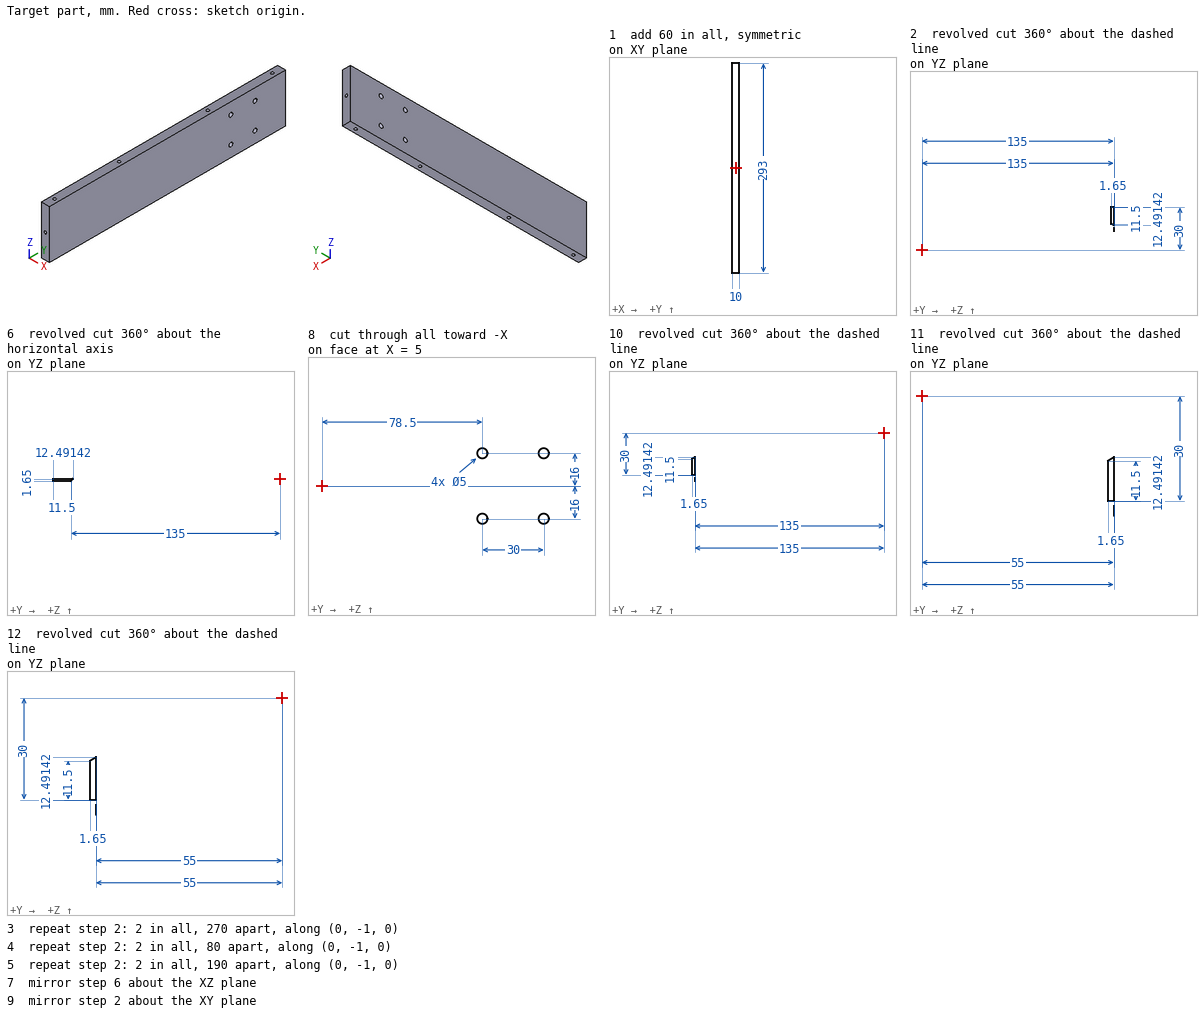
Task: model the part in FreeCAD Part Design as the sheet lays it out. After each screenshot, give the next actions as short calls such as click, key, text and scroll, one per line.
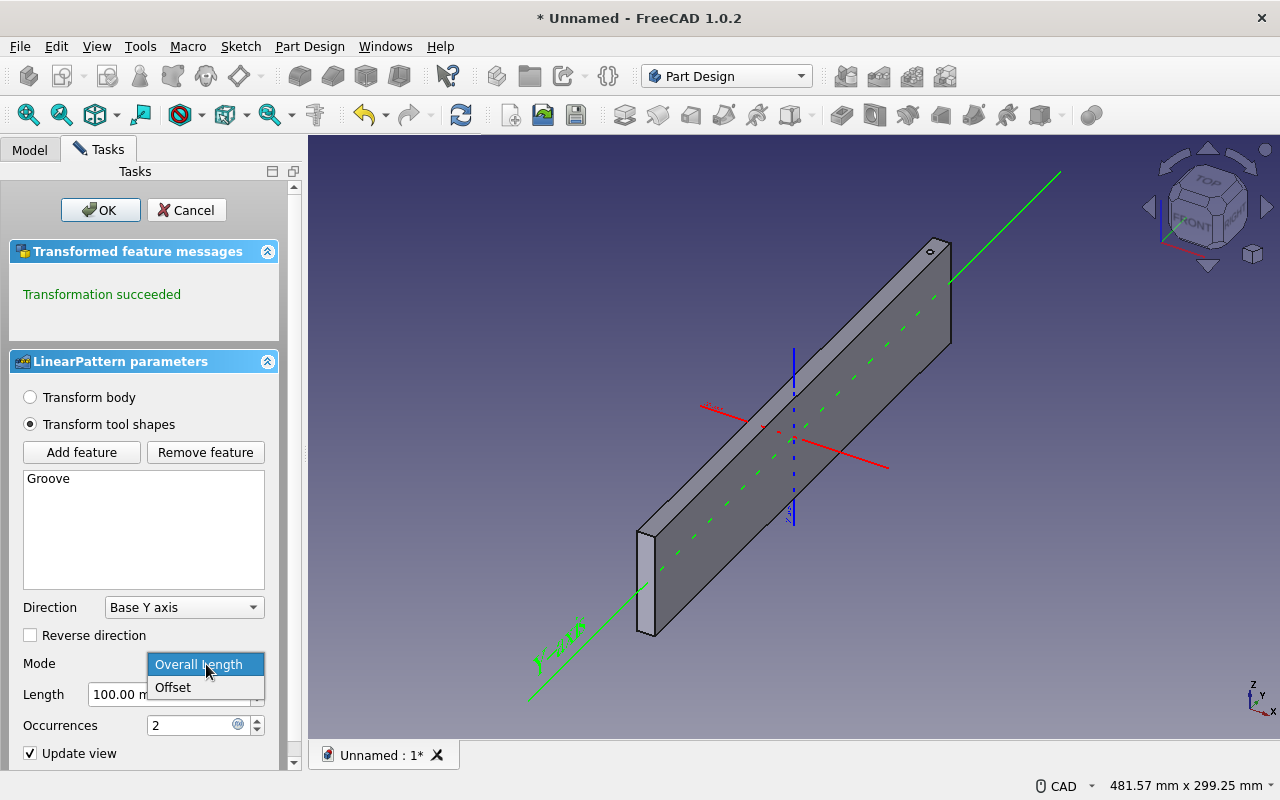
click(204, 688)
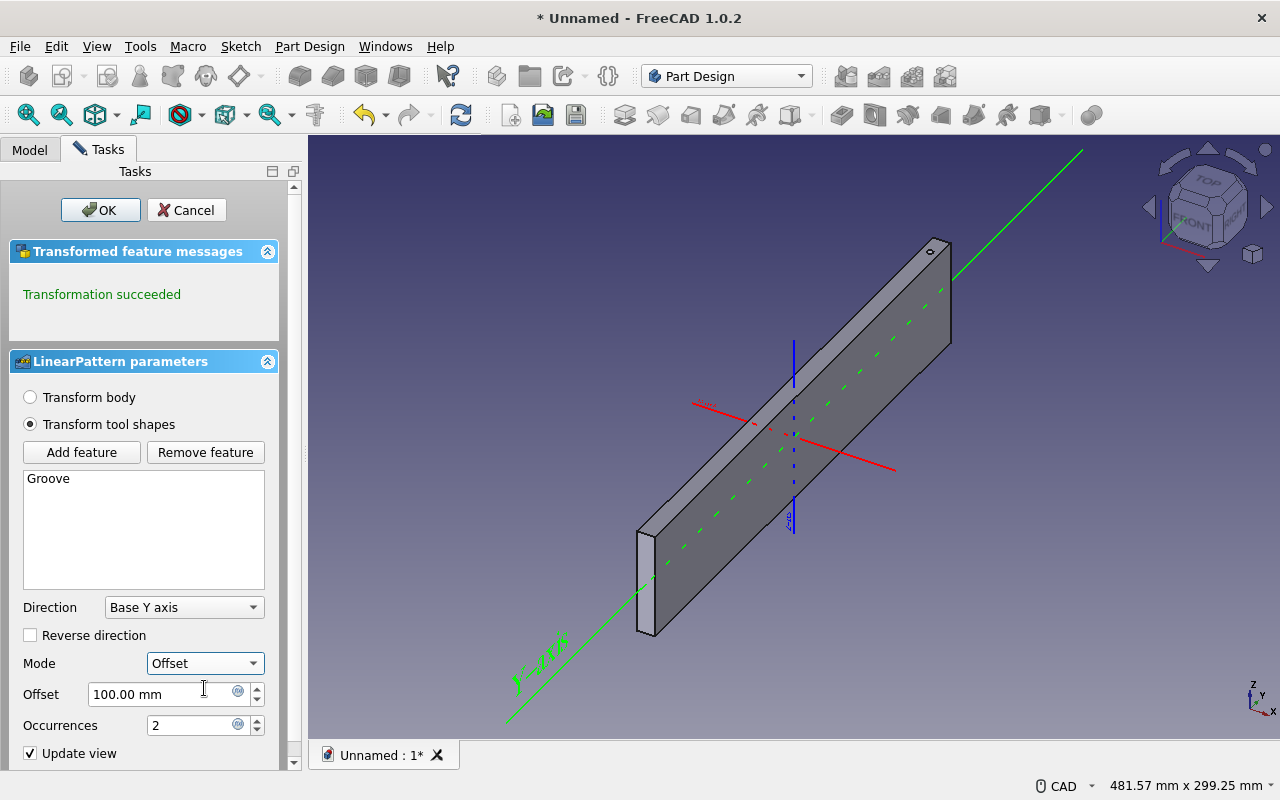
triple_click(170, 694)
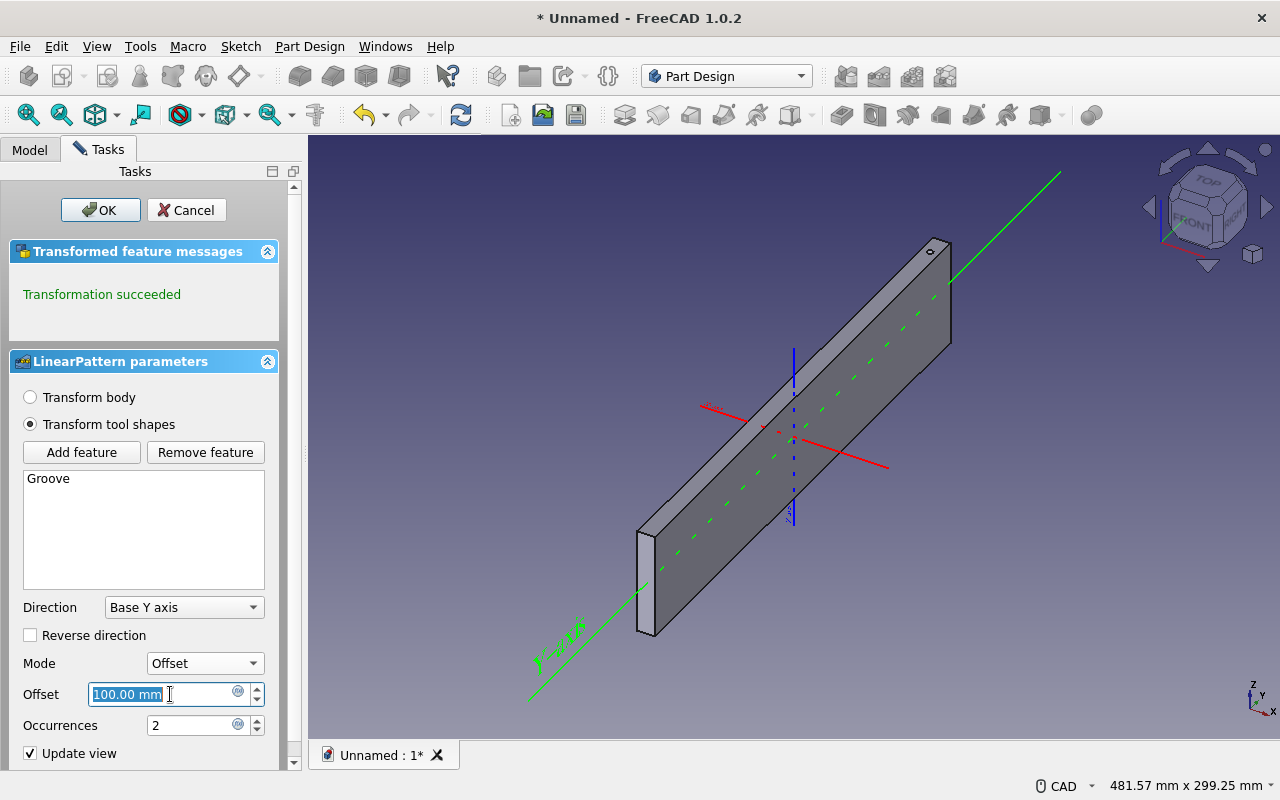
text(270)
key(Tab)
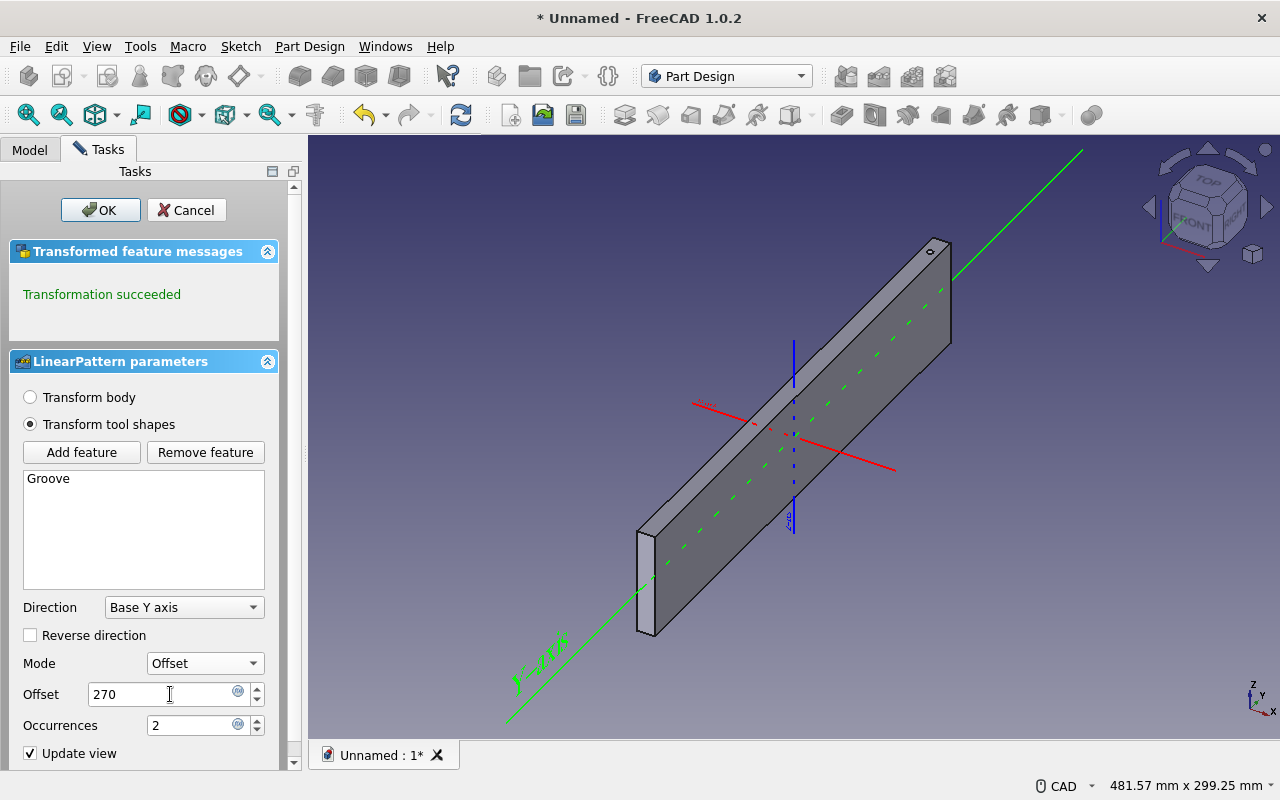
triple_click(199, 726)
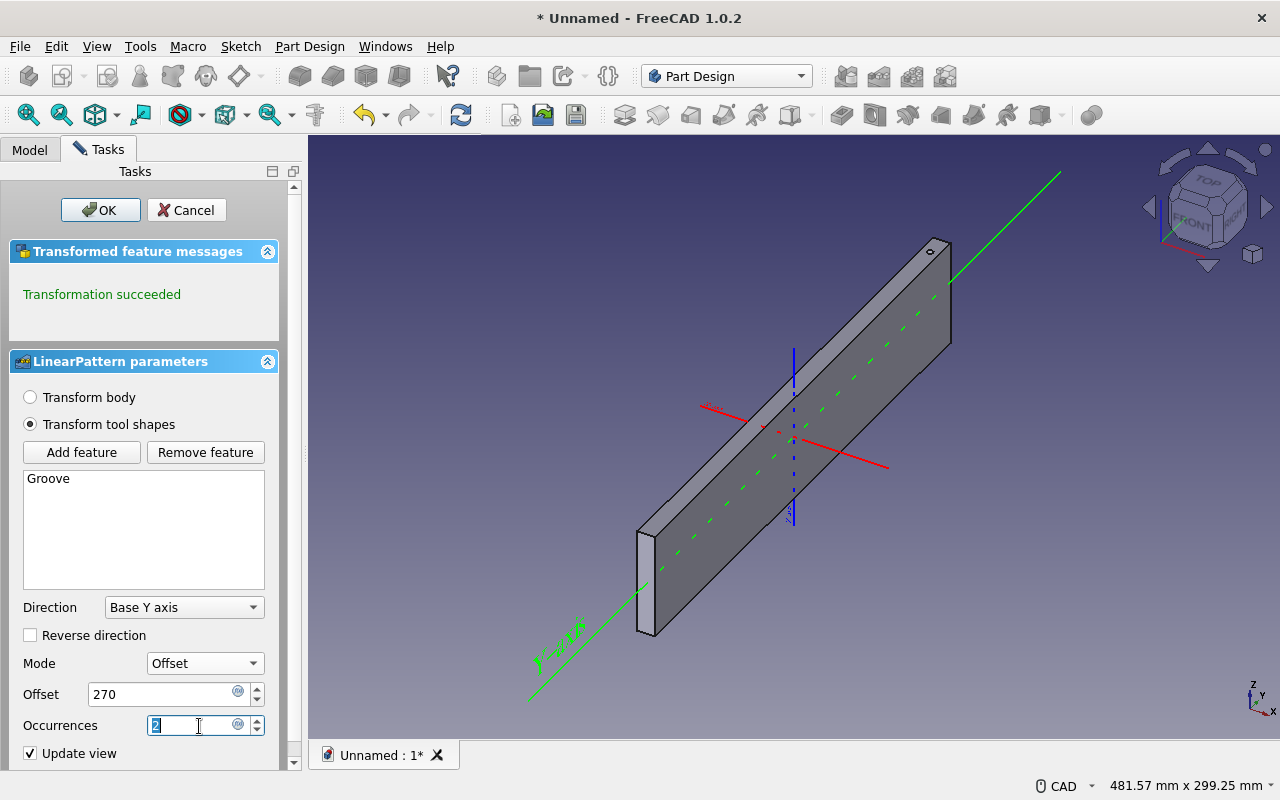
text(2)
key(Tab)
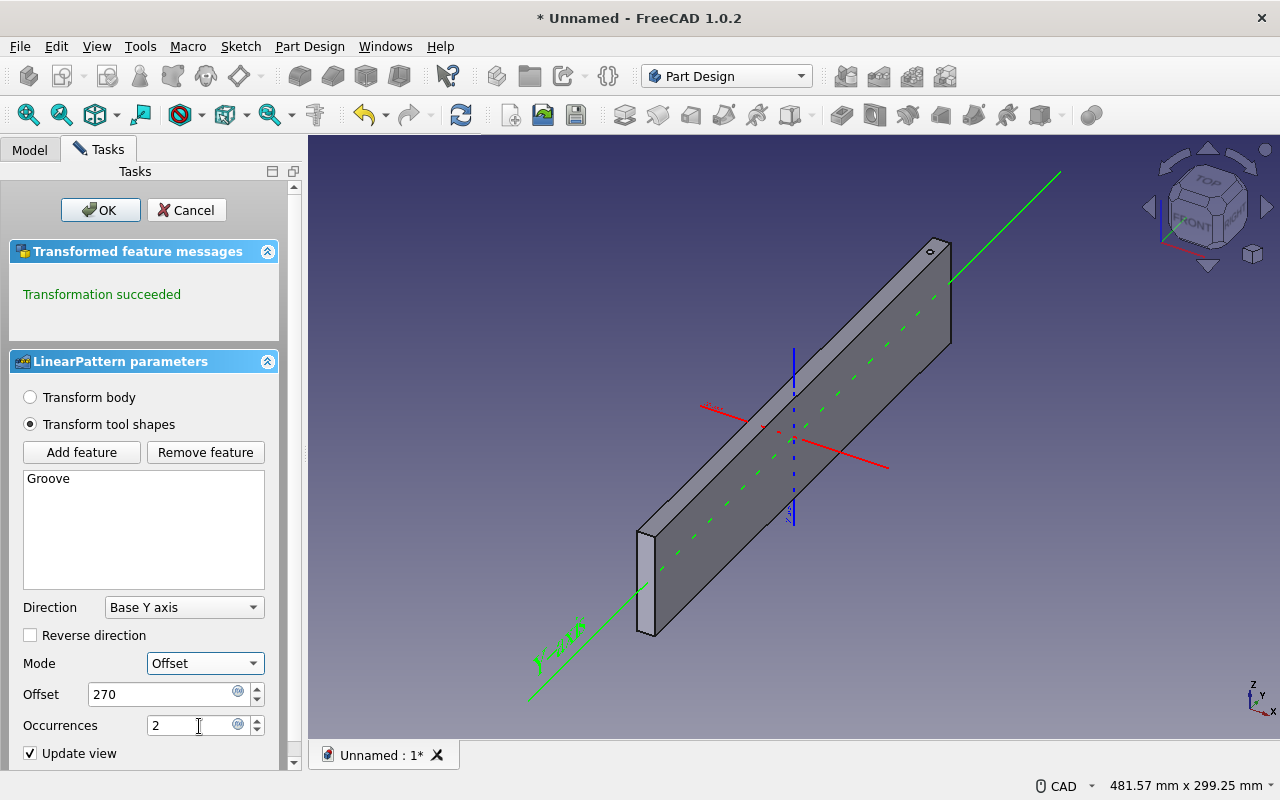
click(31, 635)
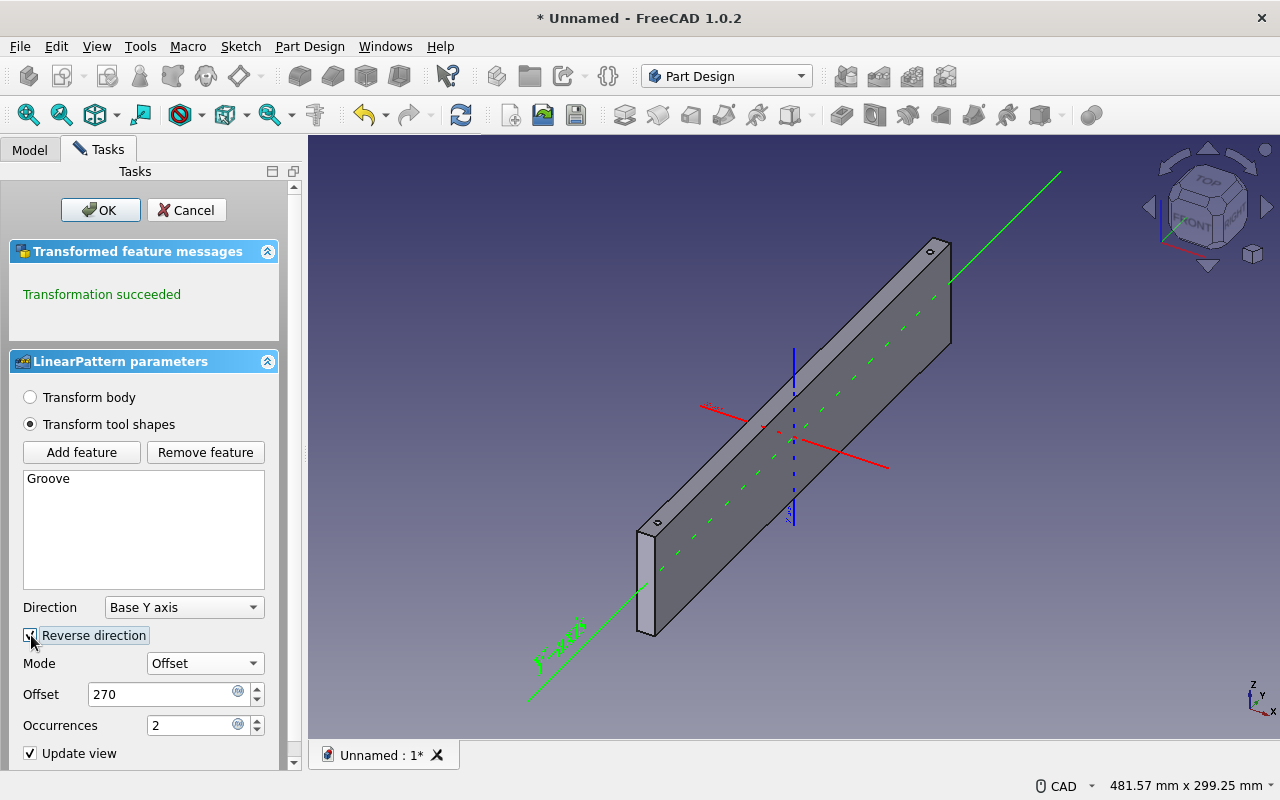
click(101, 210)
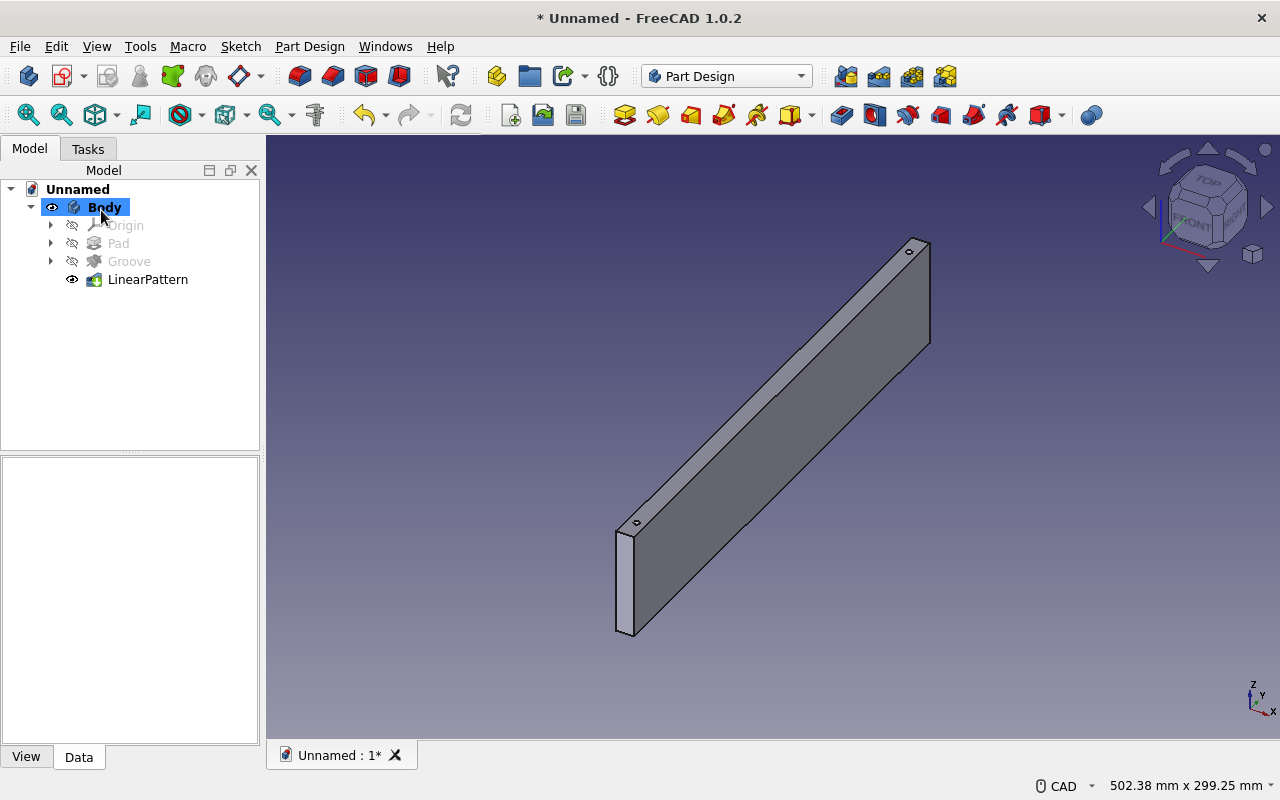
click(117, 261)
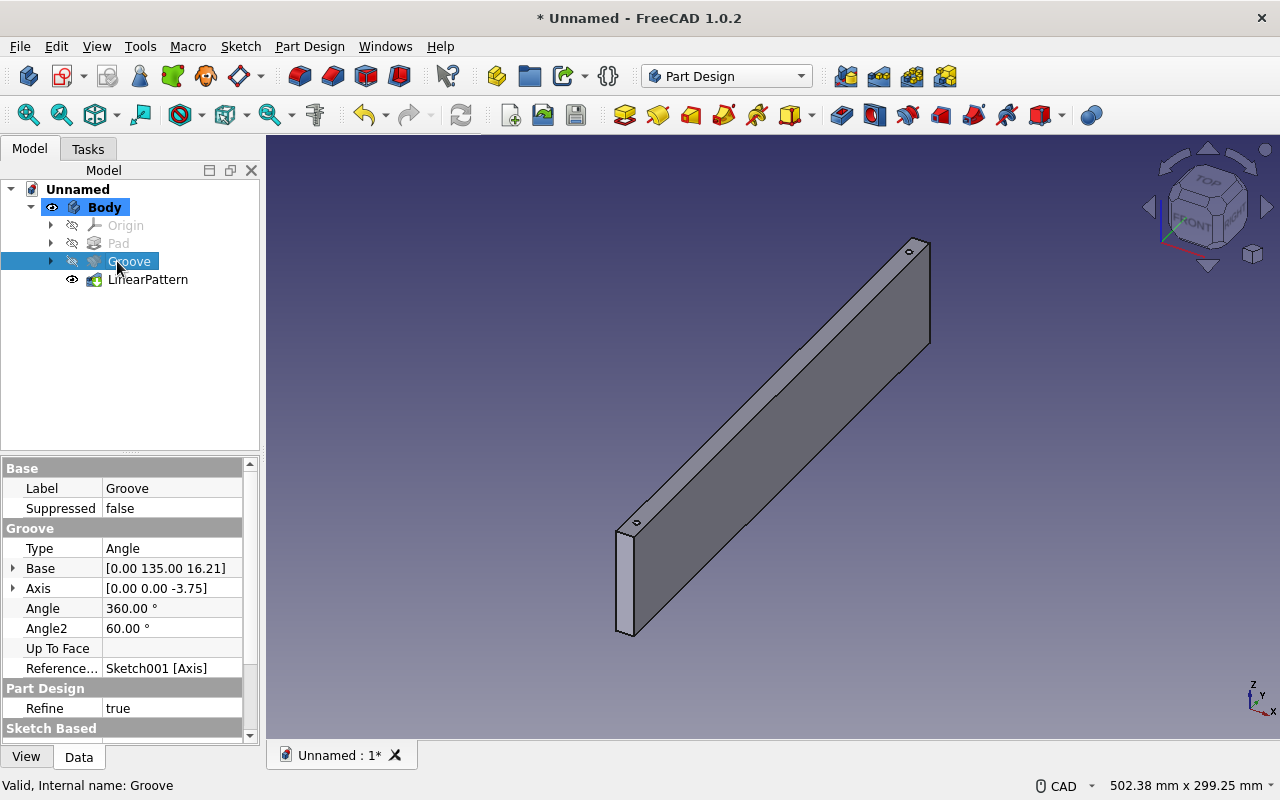
click(879, 76)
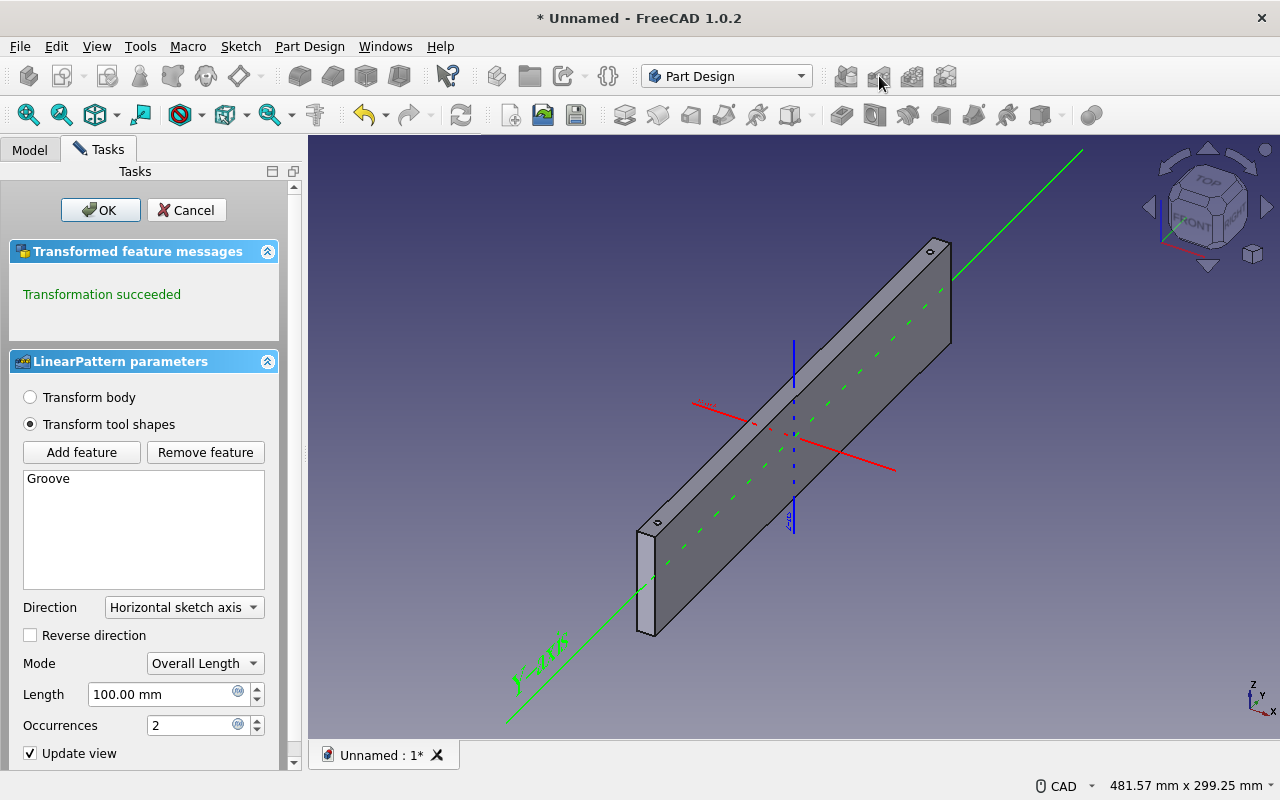
click(185, 608)